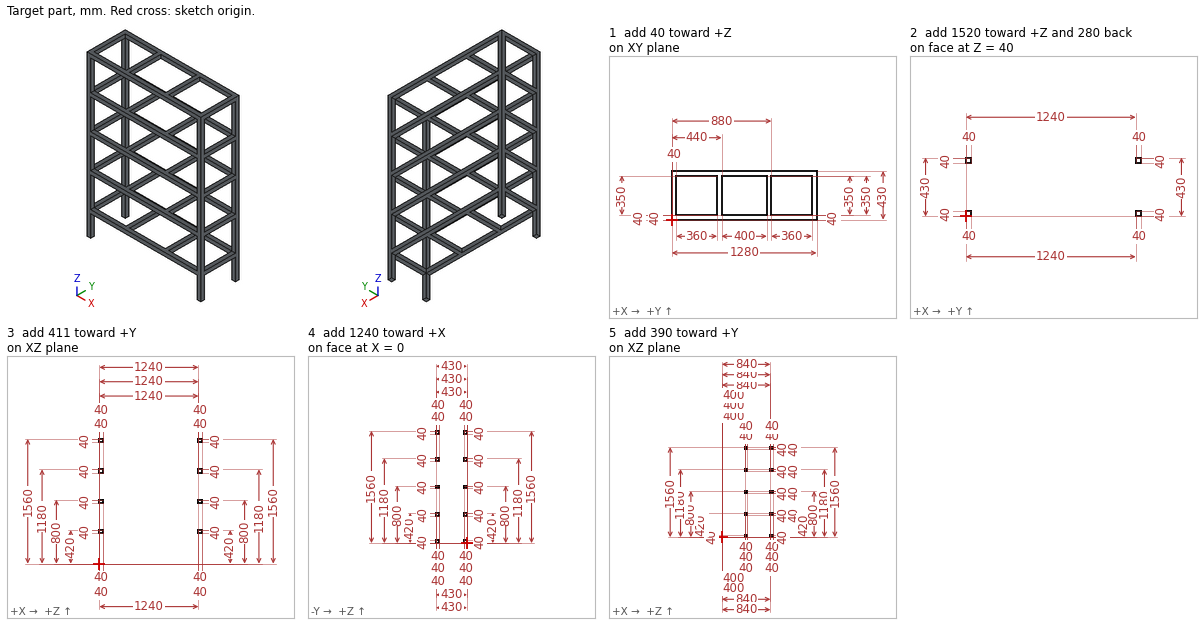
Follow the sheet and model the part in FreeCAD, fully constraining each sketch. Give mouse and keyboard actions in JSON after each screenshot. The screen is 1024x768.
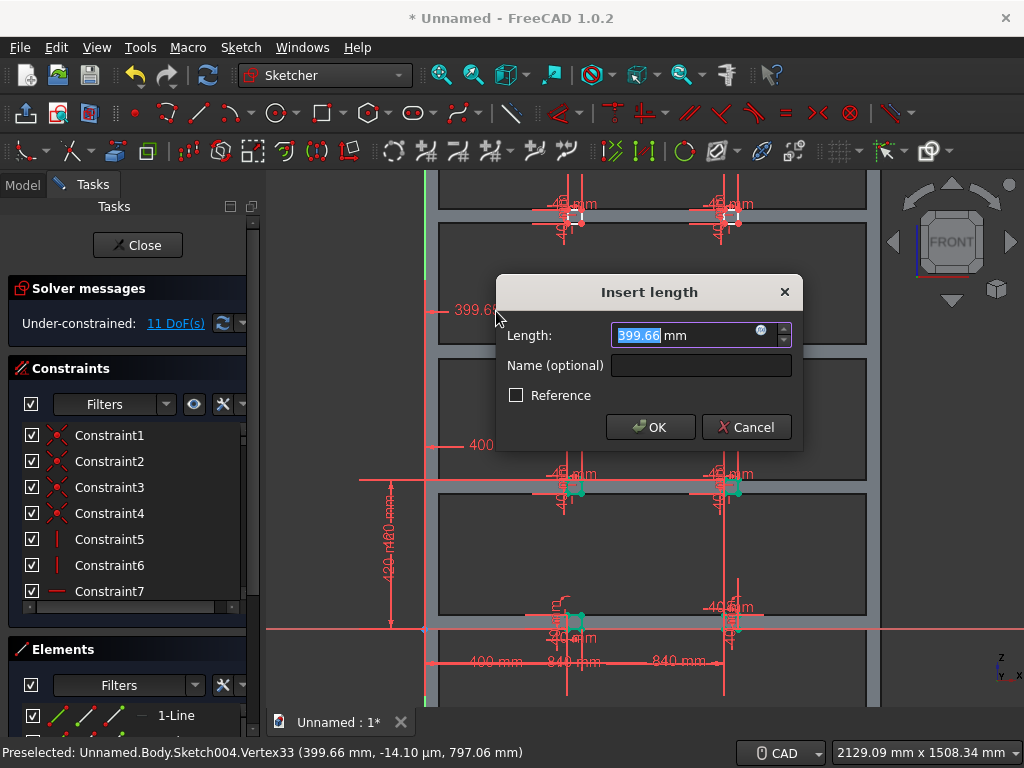
{"action": "type", "text": "400"}
{"action": "key", "text": "Return"}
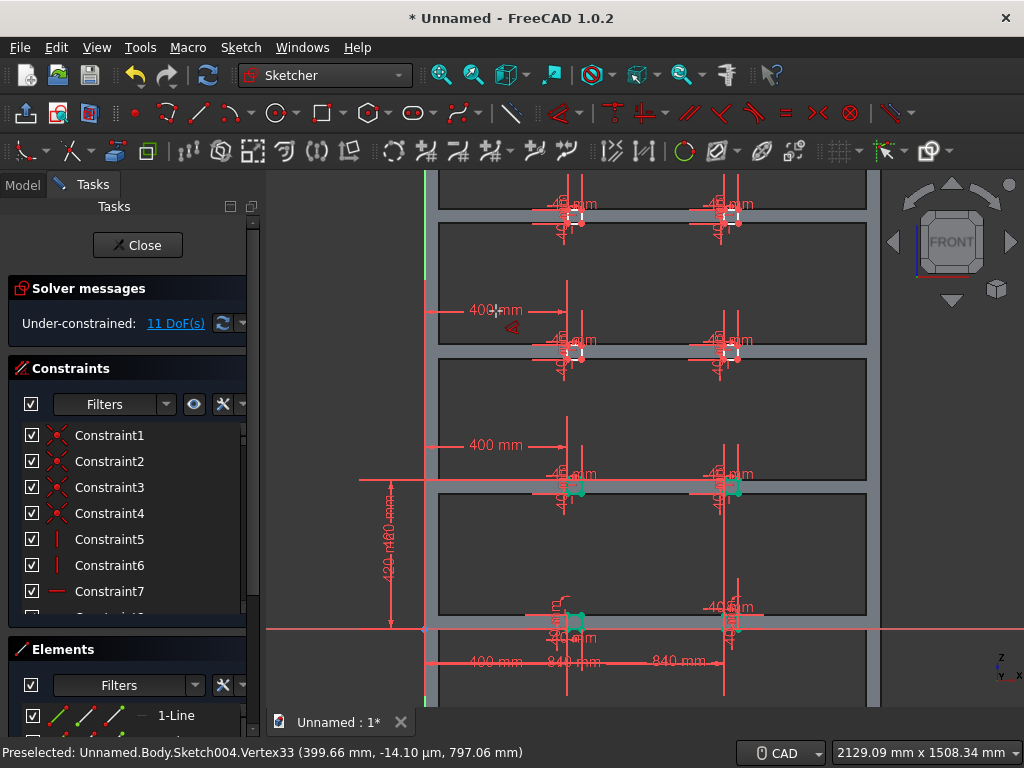
{"action": "left_click", "coordinate": [567, 345]}
{"action": "left_click", "coordinate": [391, 487]}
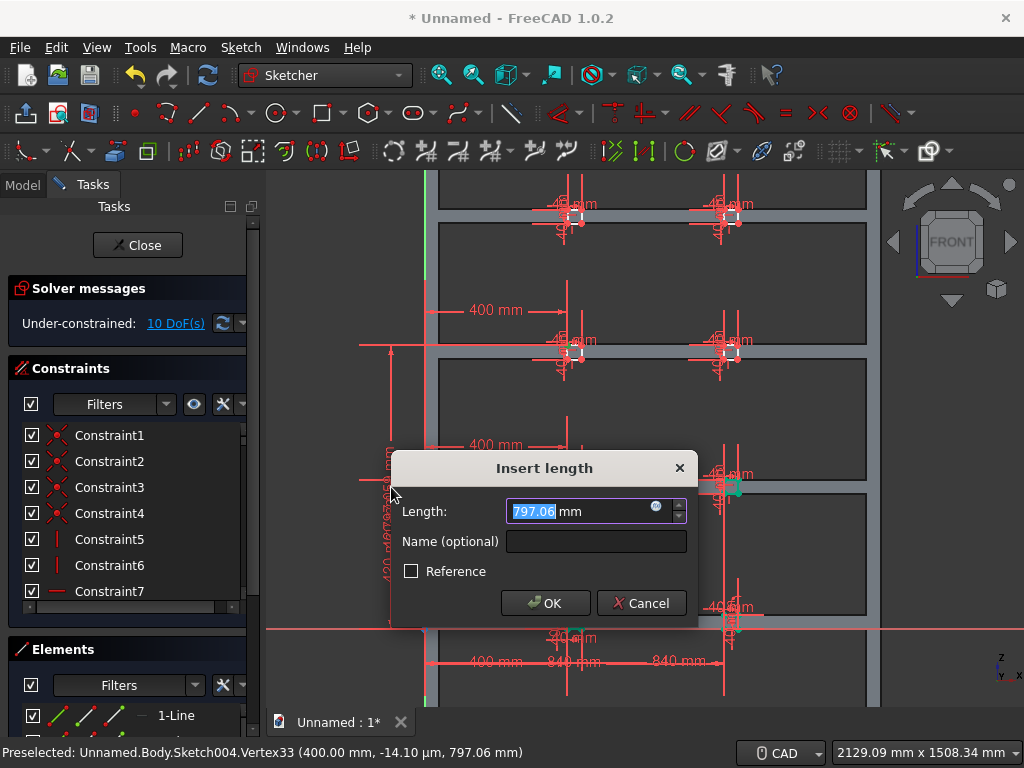
{"action": "type", "text": "800"}
{"action": "key", "text": "Return"}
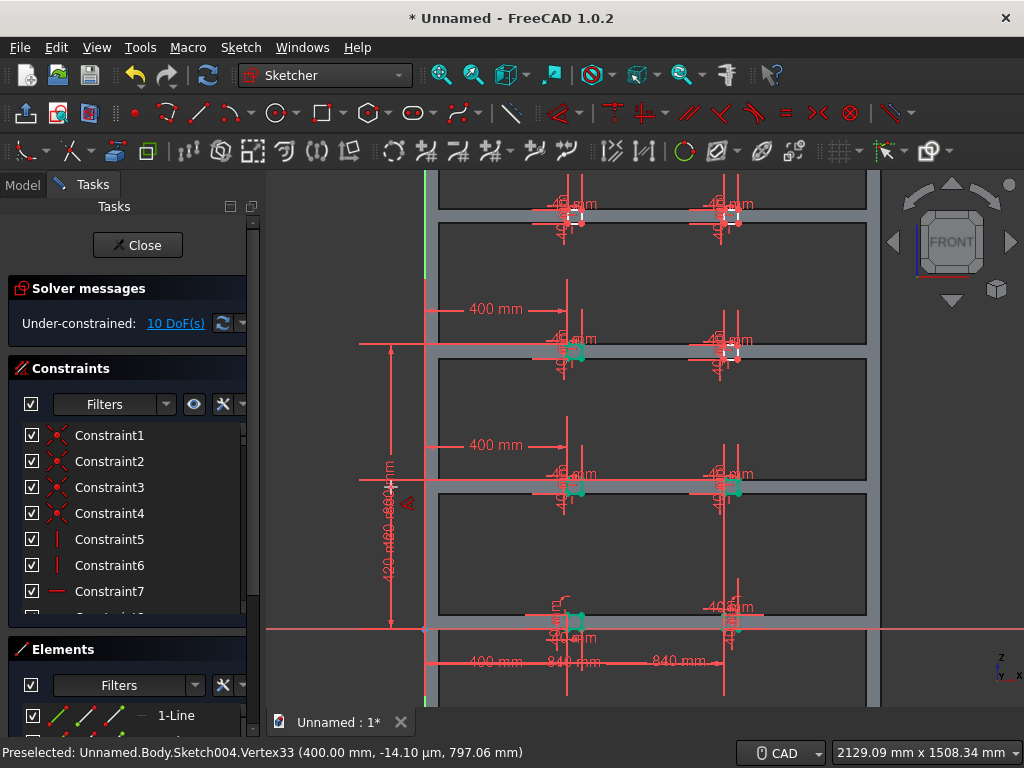
{"action": "left_click", "coordinate": [724, 345]}
{"action": "left_click", "coordinate": [574, 311]}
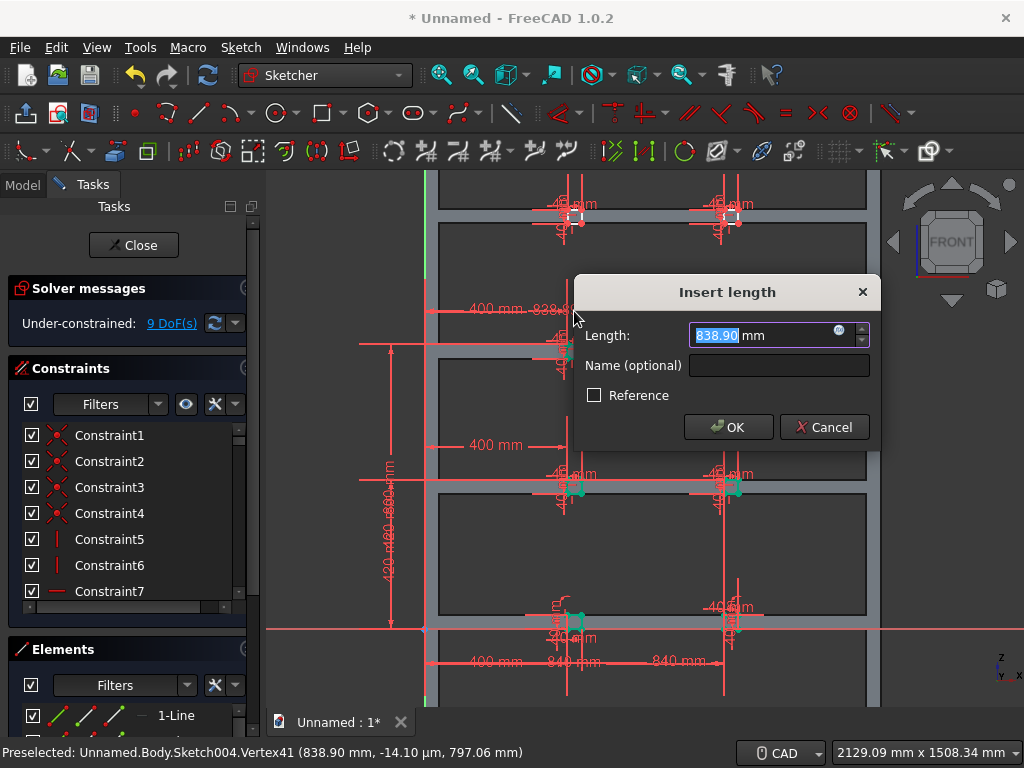
{"action": "type", "text": "840"}
{"action": "key", "text": "Return"}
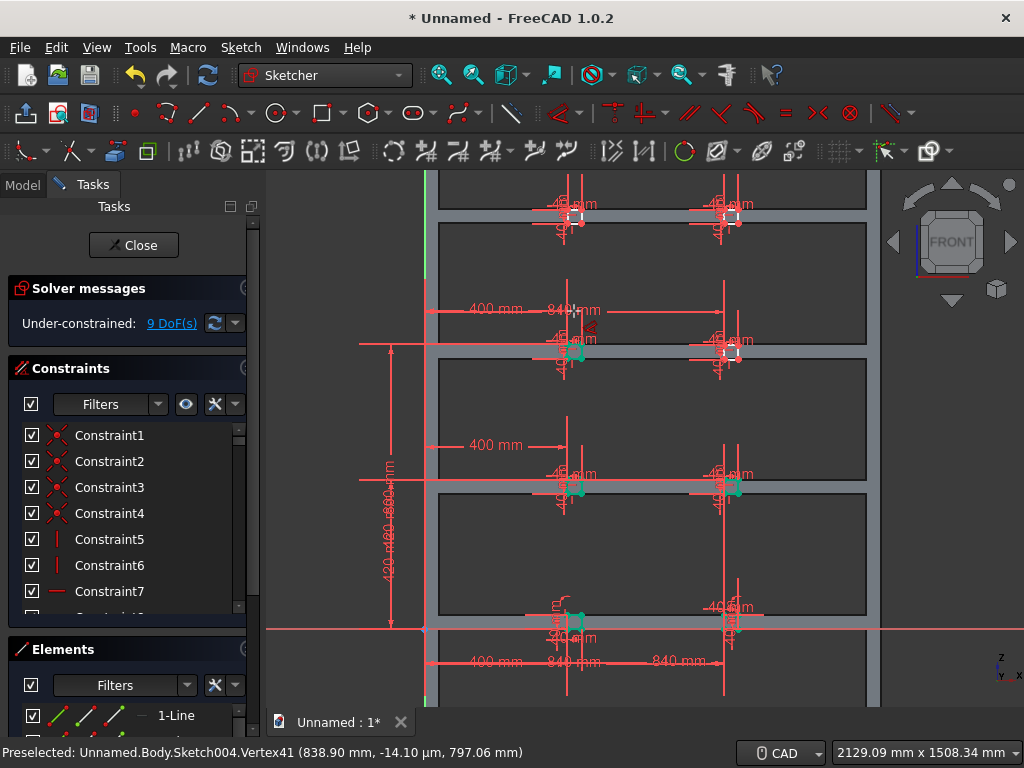
{"action": "left_click", "coordinate": [724, 345]}
{"action": "left_click", "coordinate": [391, 422]}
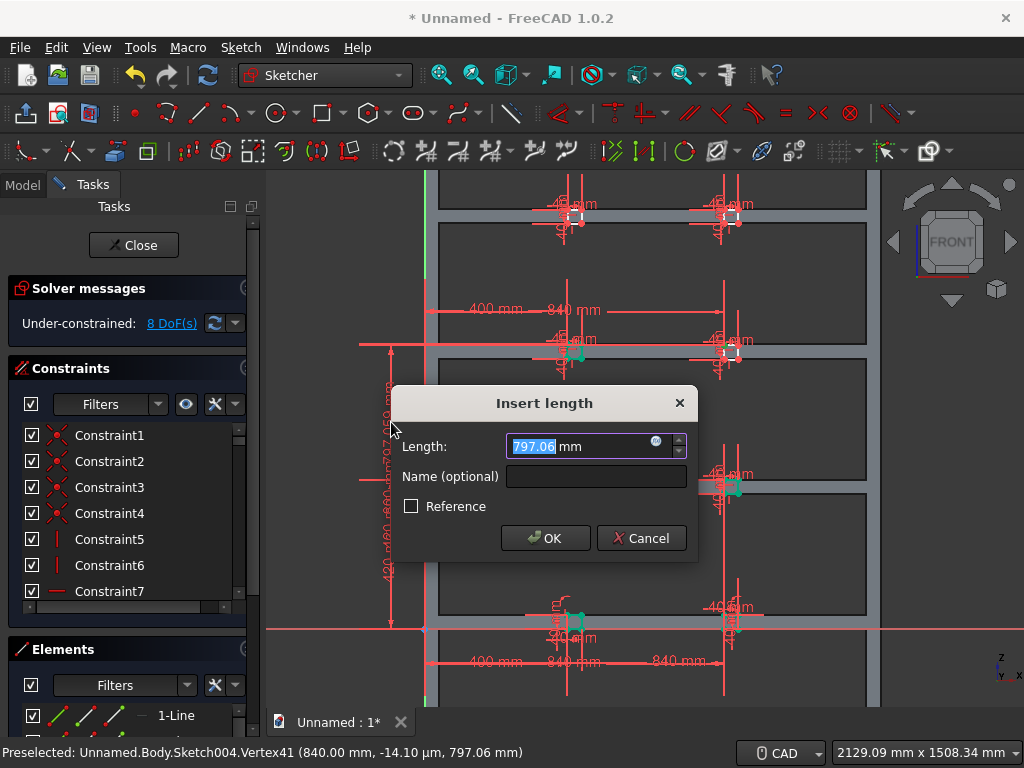
{"action": "type", "text": "800"}
{"action": "key", "text": "Return"}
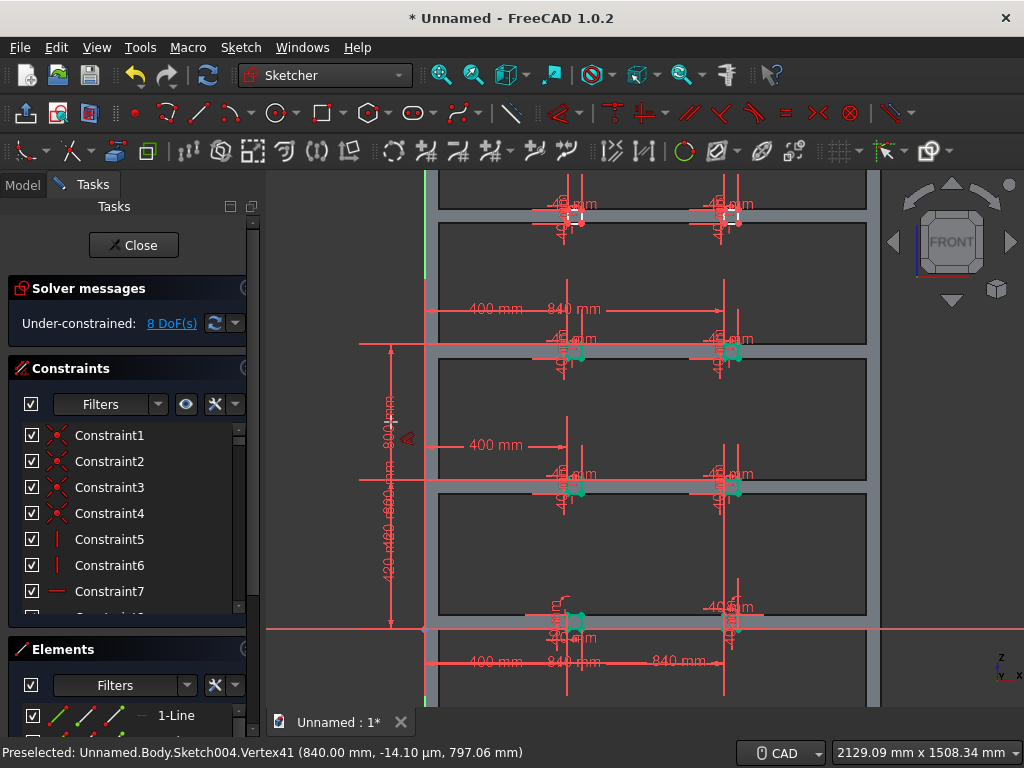
{"action": "left_click", "coordinate": [568, 210]}
{"action": "left_click", "coordinate": [446, 663]}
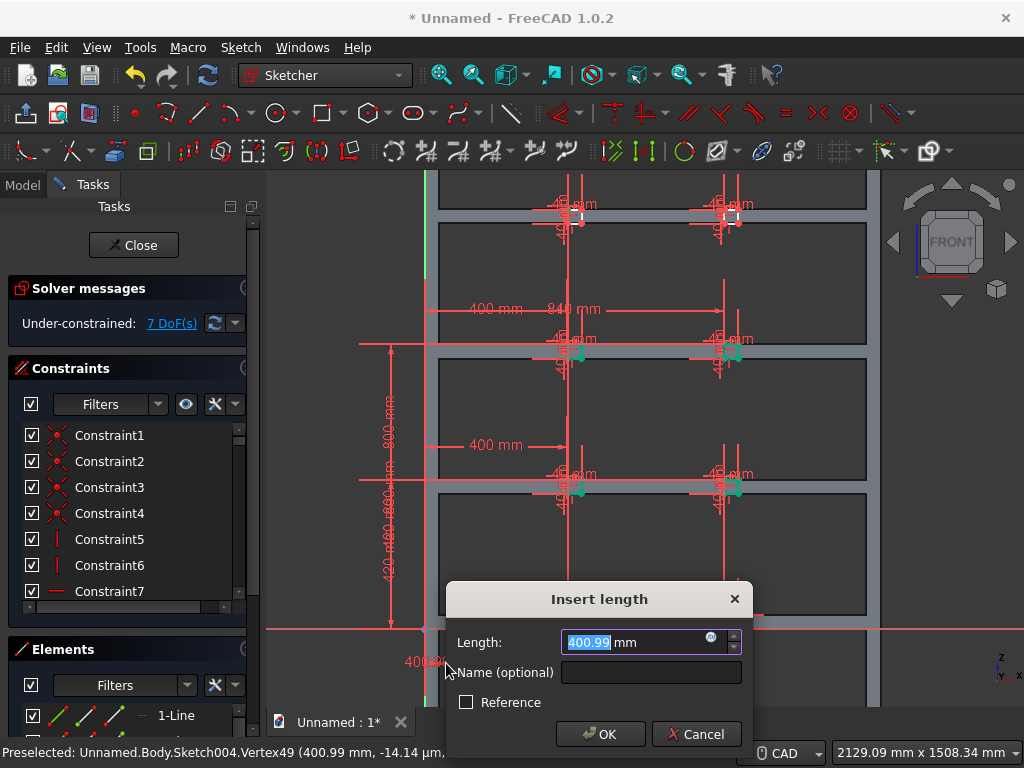
{"action": "type", "text": "400"}
{"action": "key", "text": "Return"}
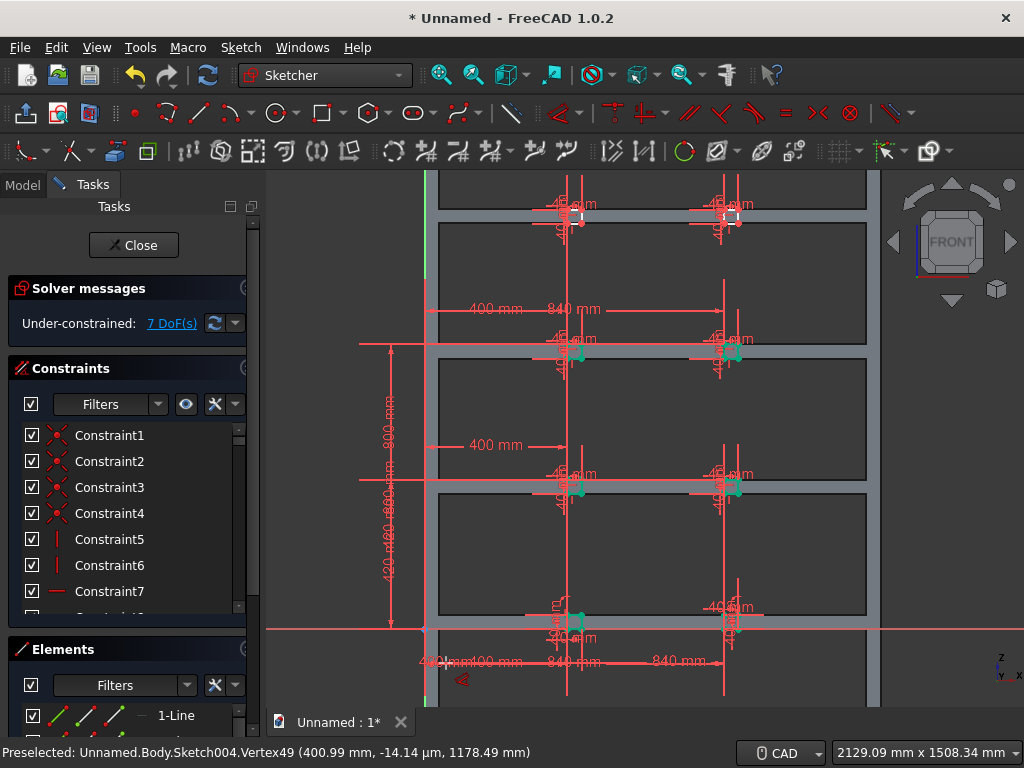
{"action": "left_click", "coordinate": [724, 210]}
{"action": "left_click", "coordinate": [643, 663]}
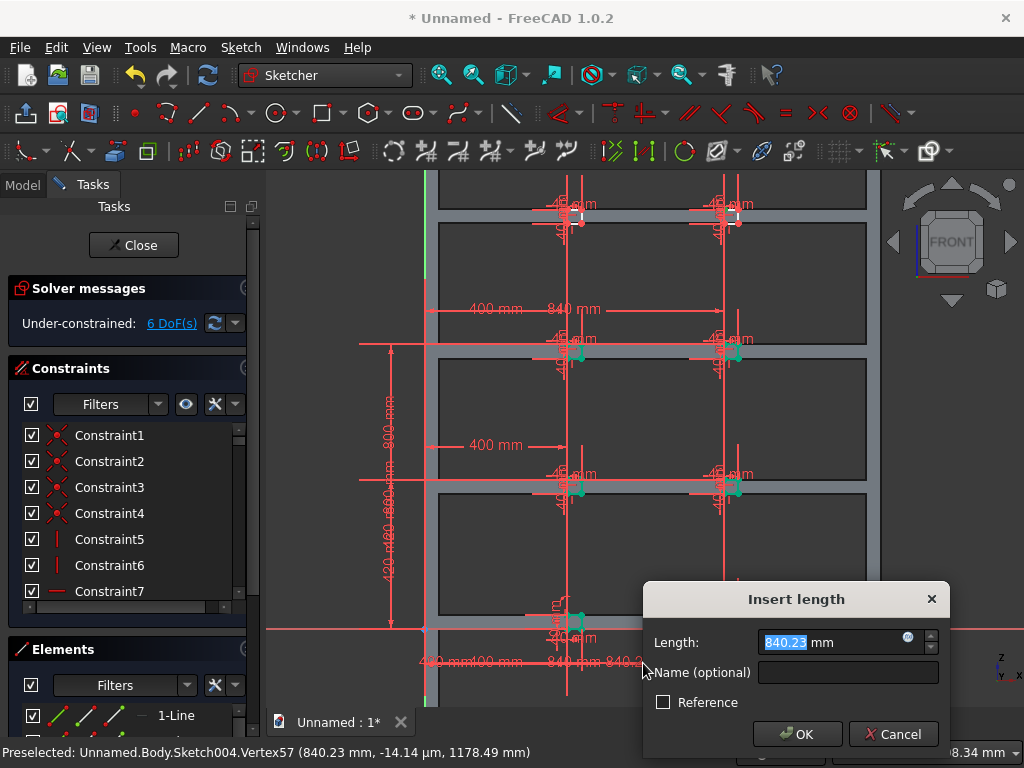
{"action": "type", "text": "840"}
{"action": "key", "text": "Return"}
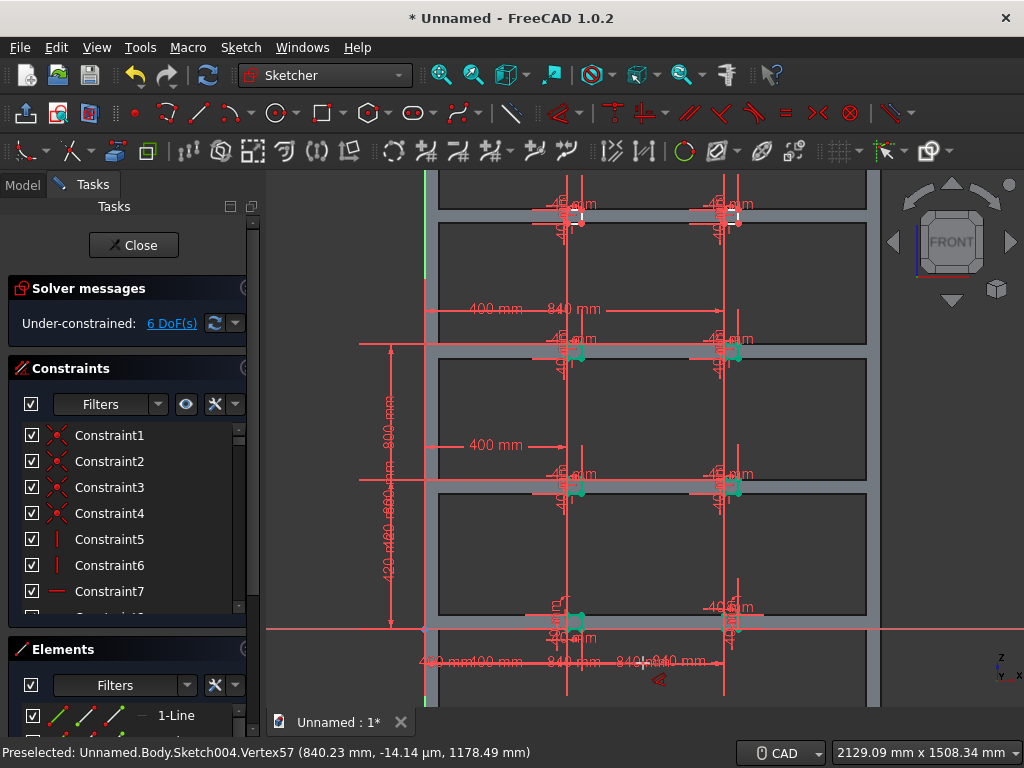
{"action": "scroll", "coordinate": [566, 615], "scroll_direction": "down", "scroll_amount": 2}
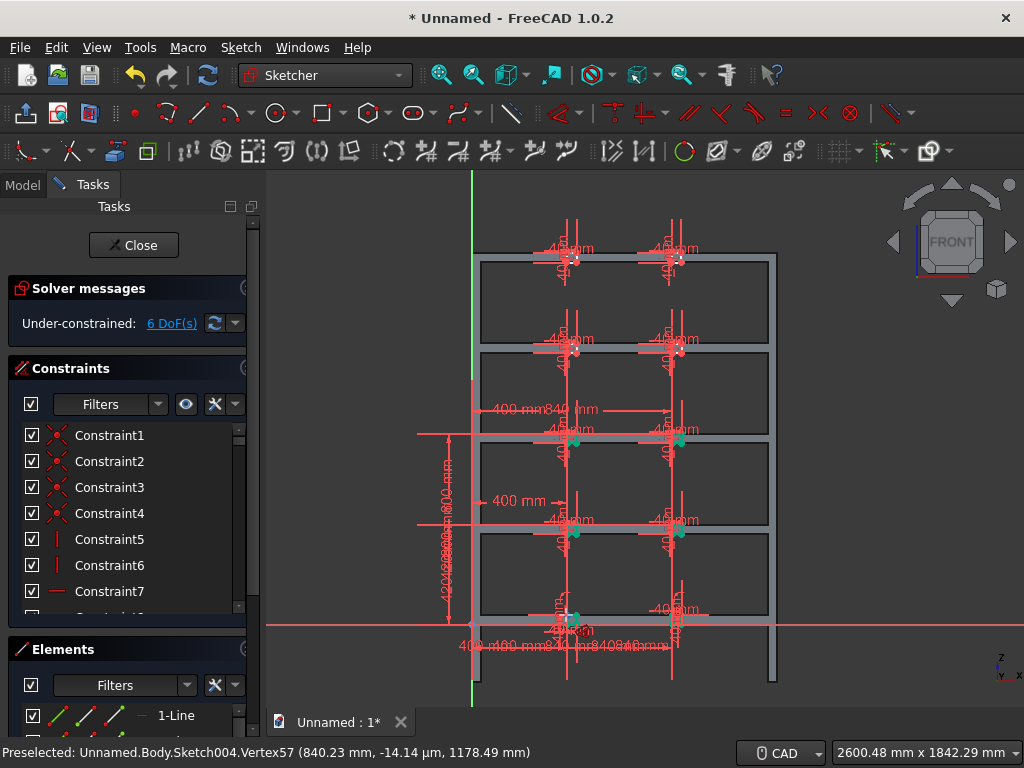
{"action": "scroll", "coordinate": [672, 253], "scroll_direction": "up", "scroll_amount": 2}